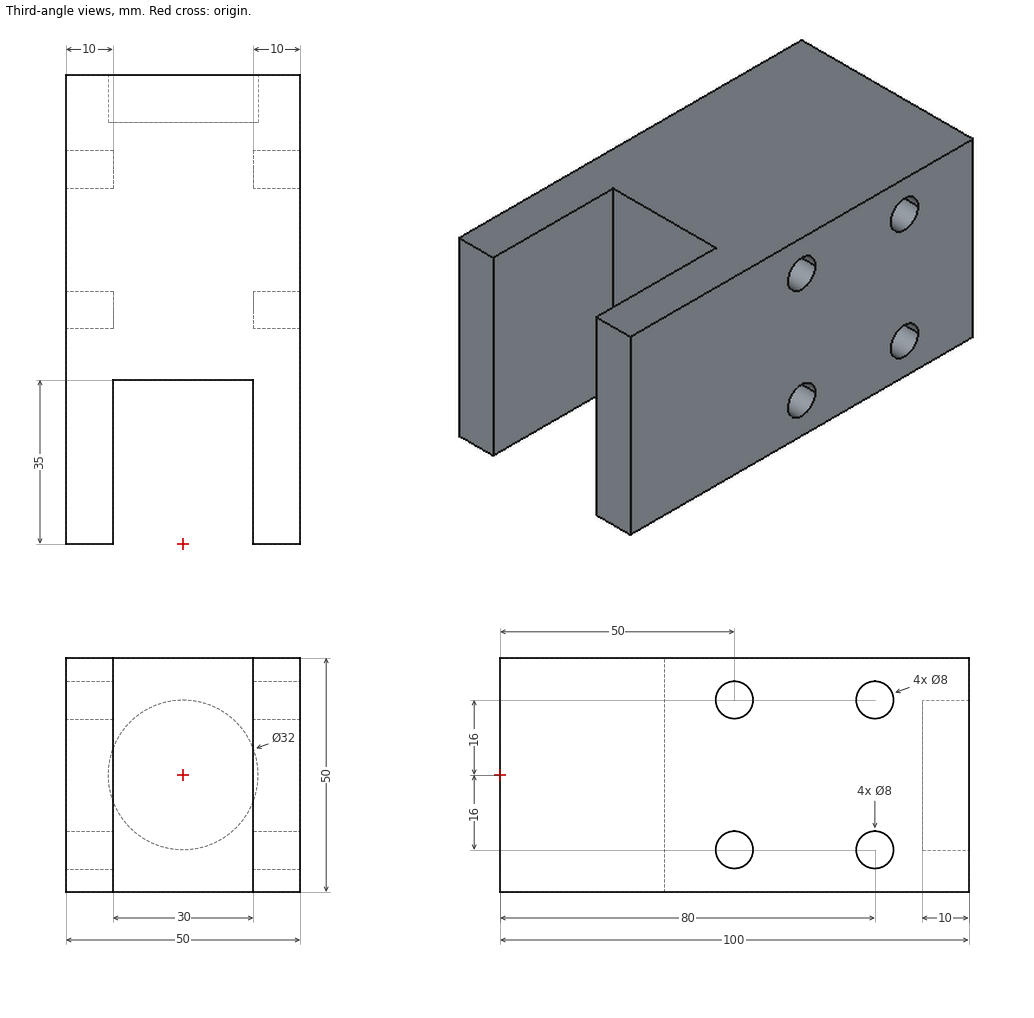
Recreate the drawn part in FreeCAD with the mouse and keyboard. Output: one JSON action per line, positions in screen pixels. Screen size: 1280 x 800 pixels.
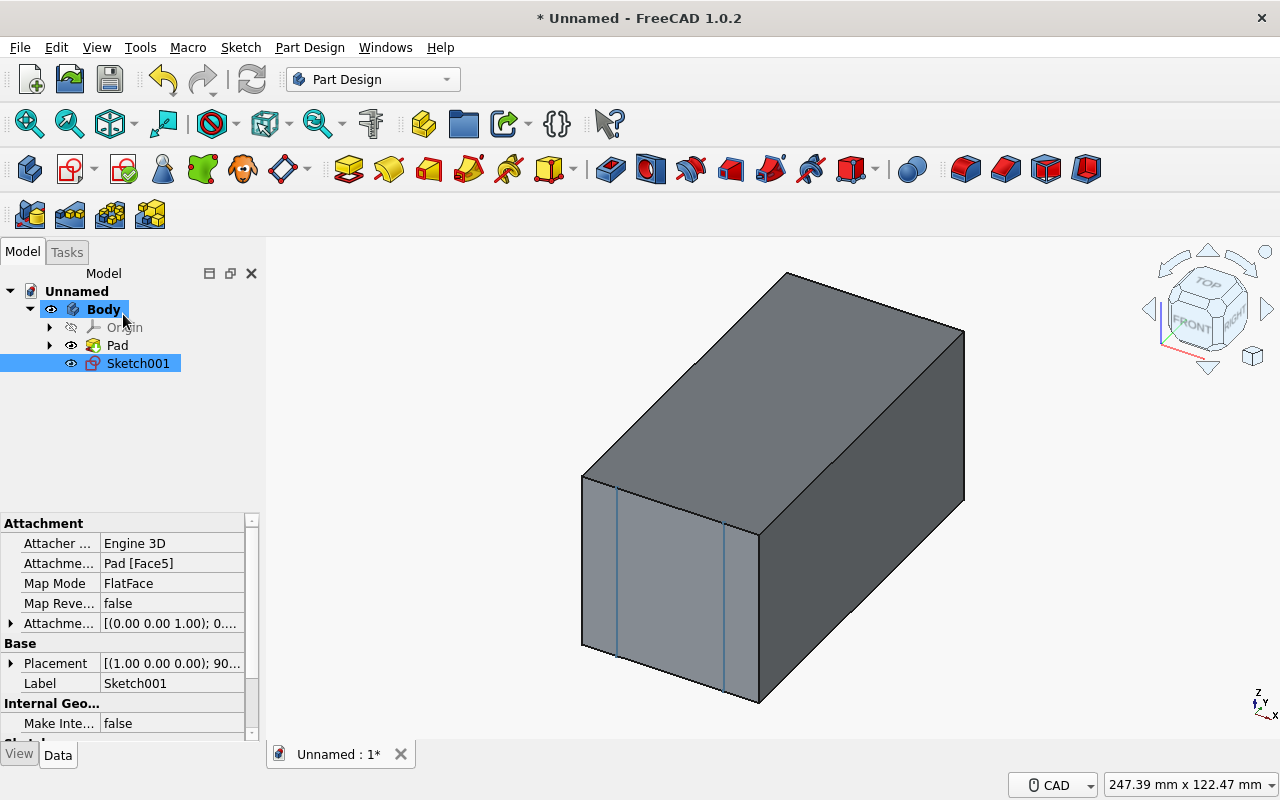
{"action": "left_click", "coordinate": [612, 170]}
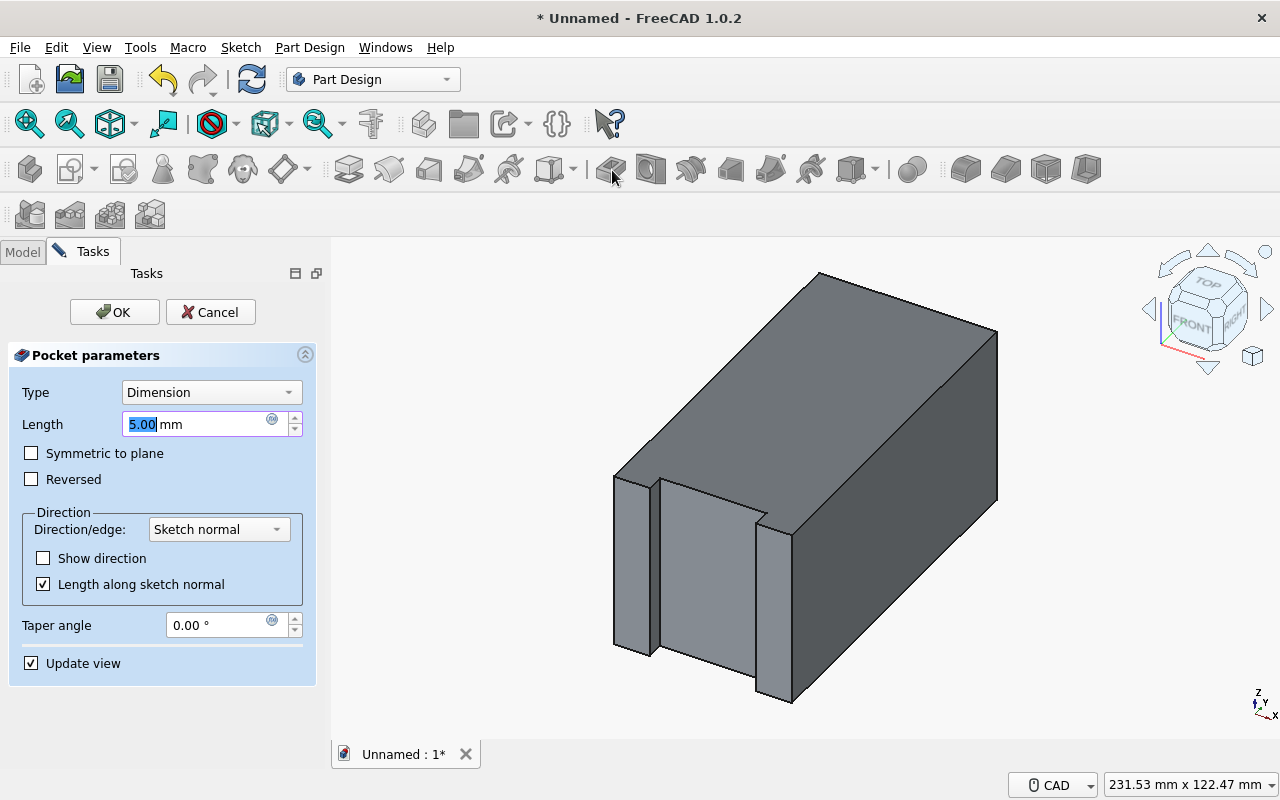
{"action": "type", "text": "35"}
{"action": "key", "text": "Tab"}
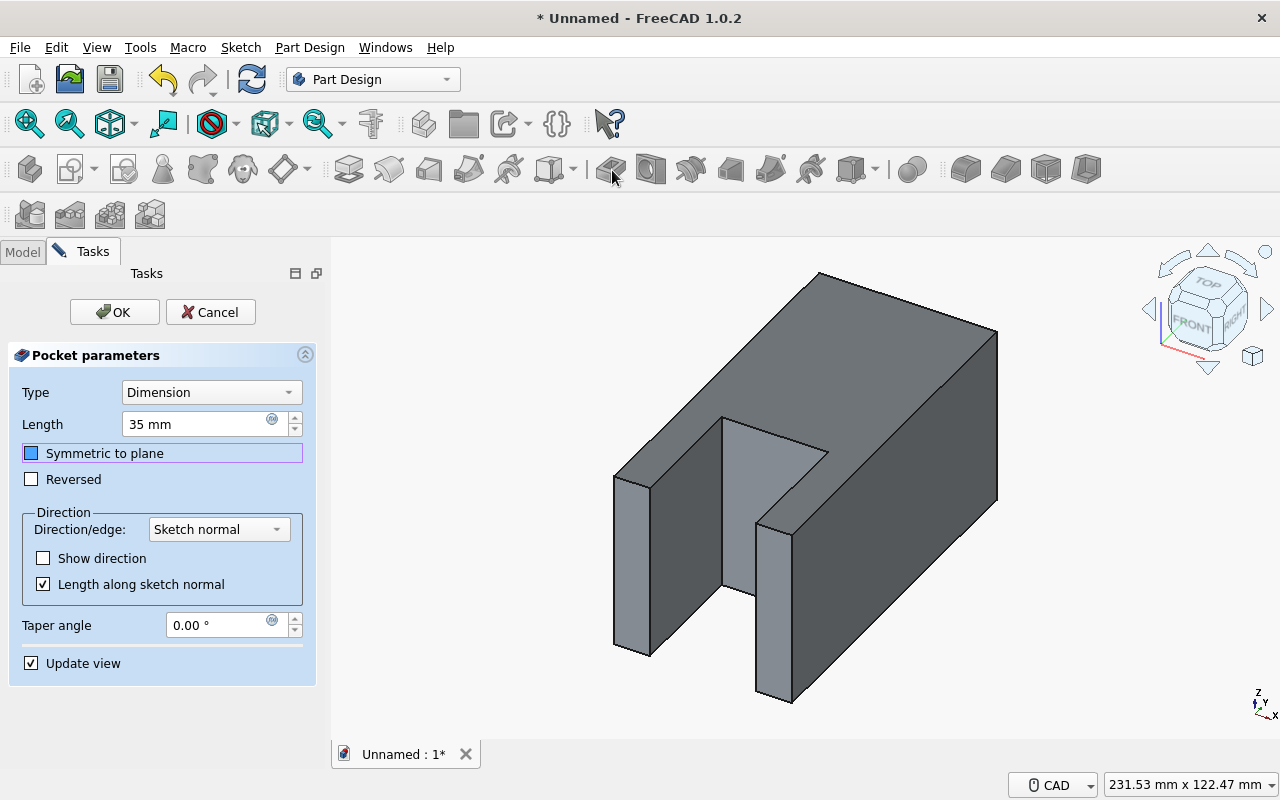
{"action": "left_click", "coordinate": [115, 312]}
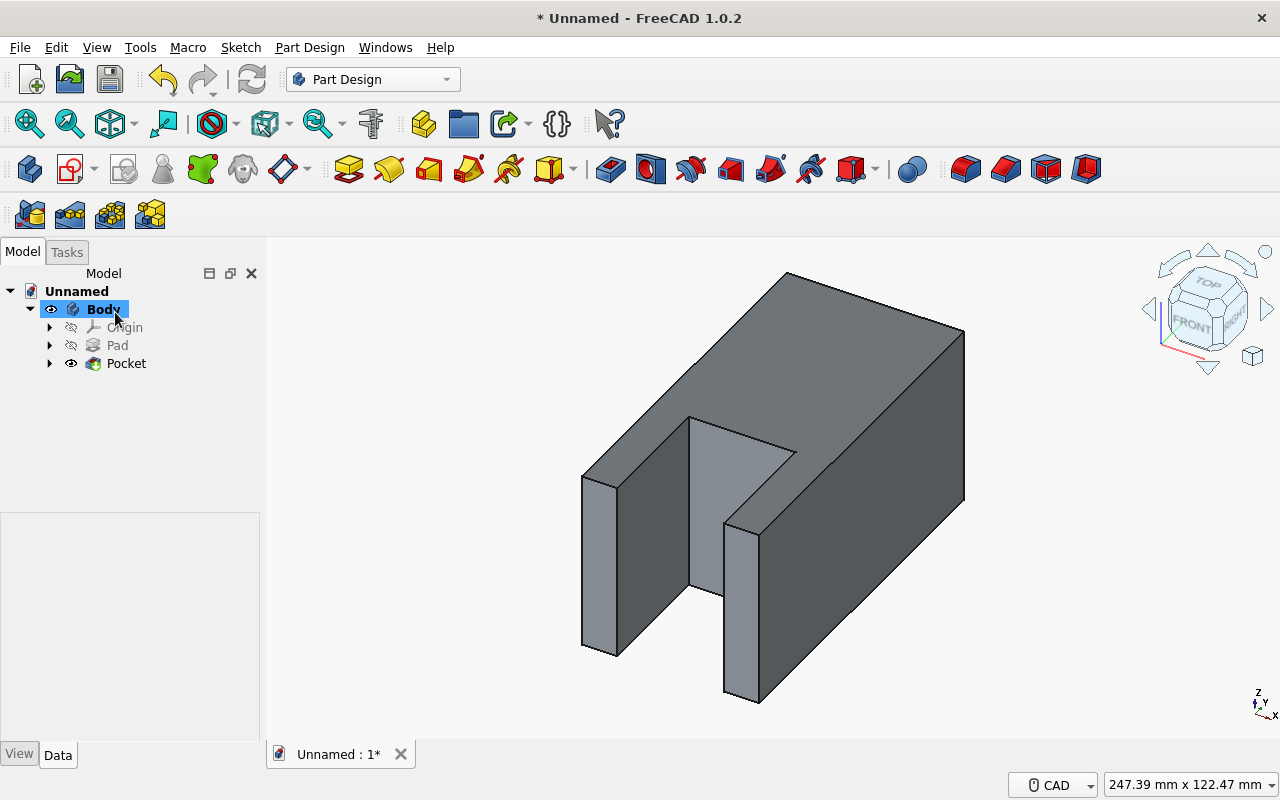
{"action": "key", "text": "4"}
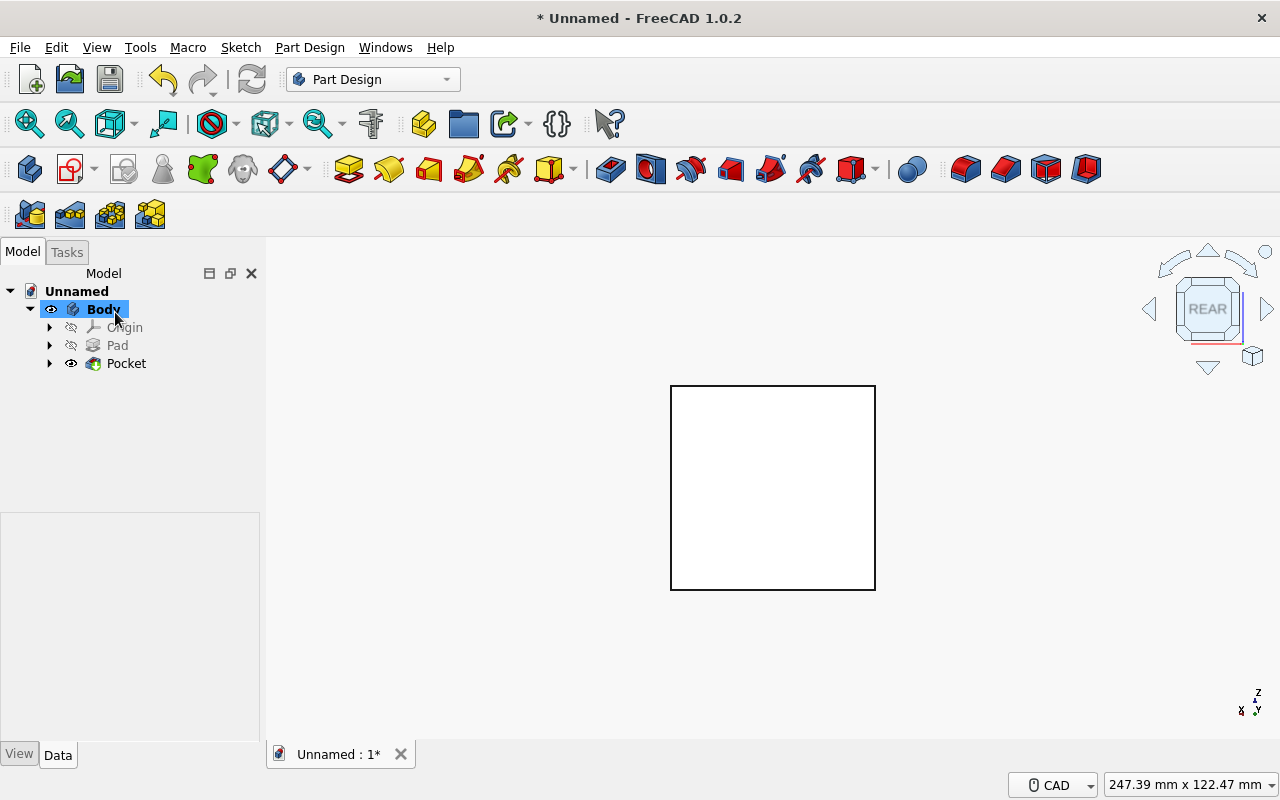
{"action": "left_click", "coordinate": [30, 124]}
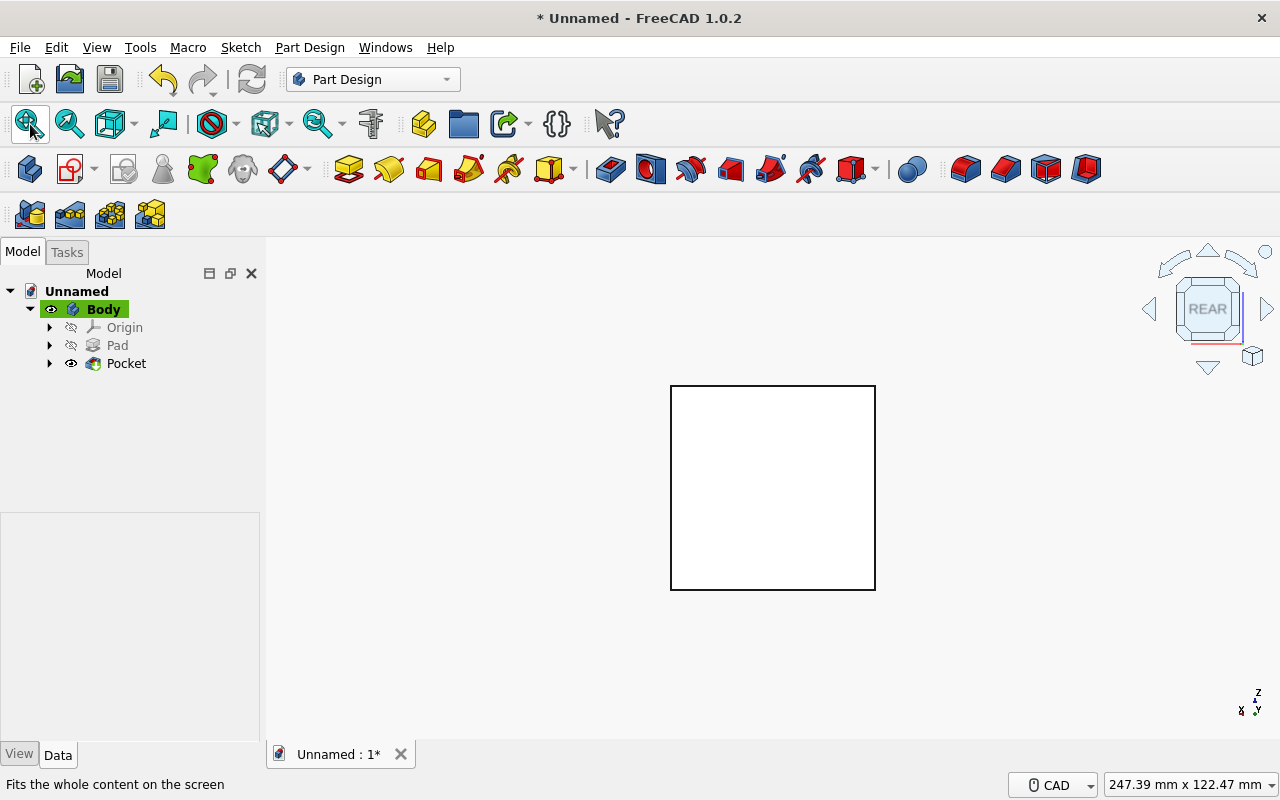
{"action": "left_click", "coordinate": [773, 487]}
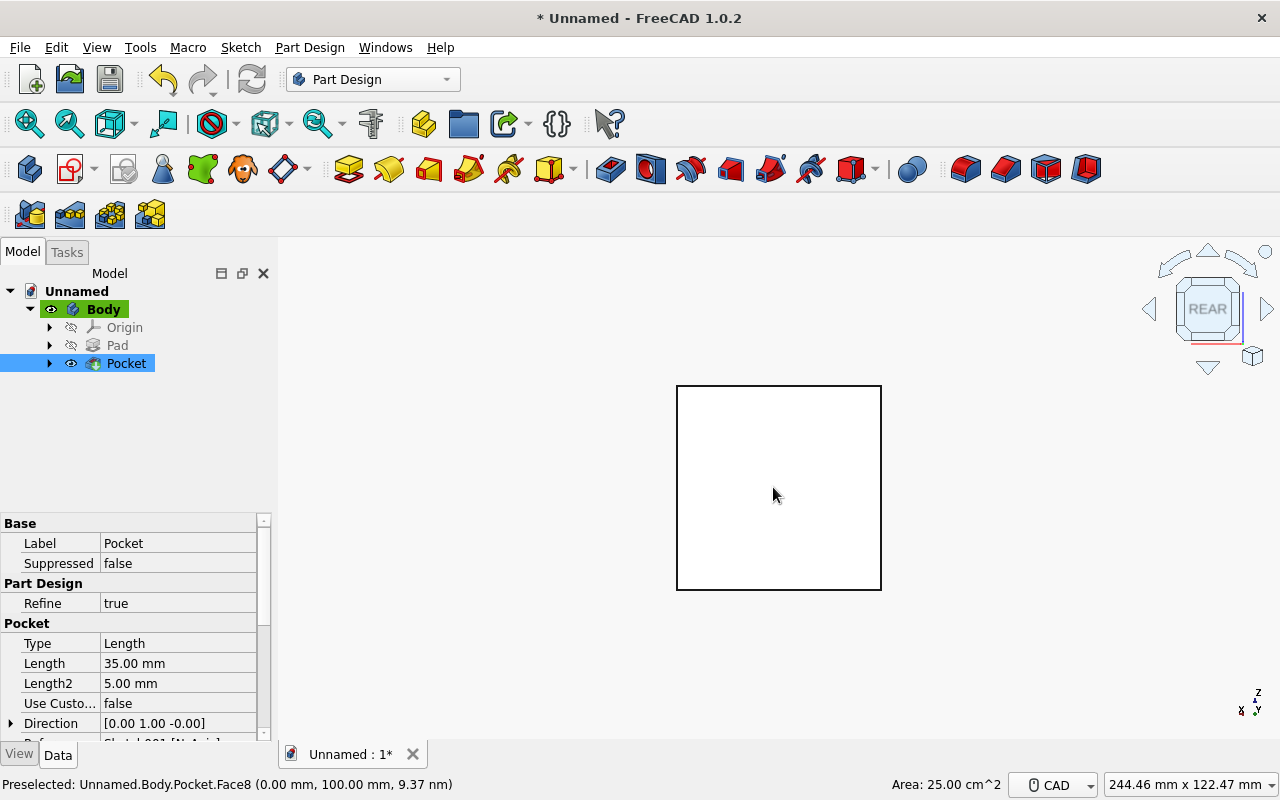
{"action": "left_click", "coordinate": [70, 170]}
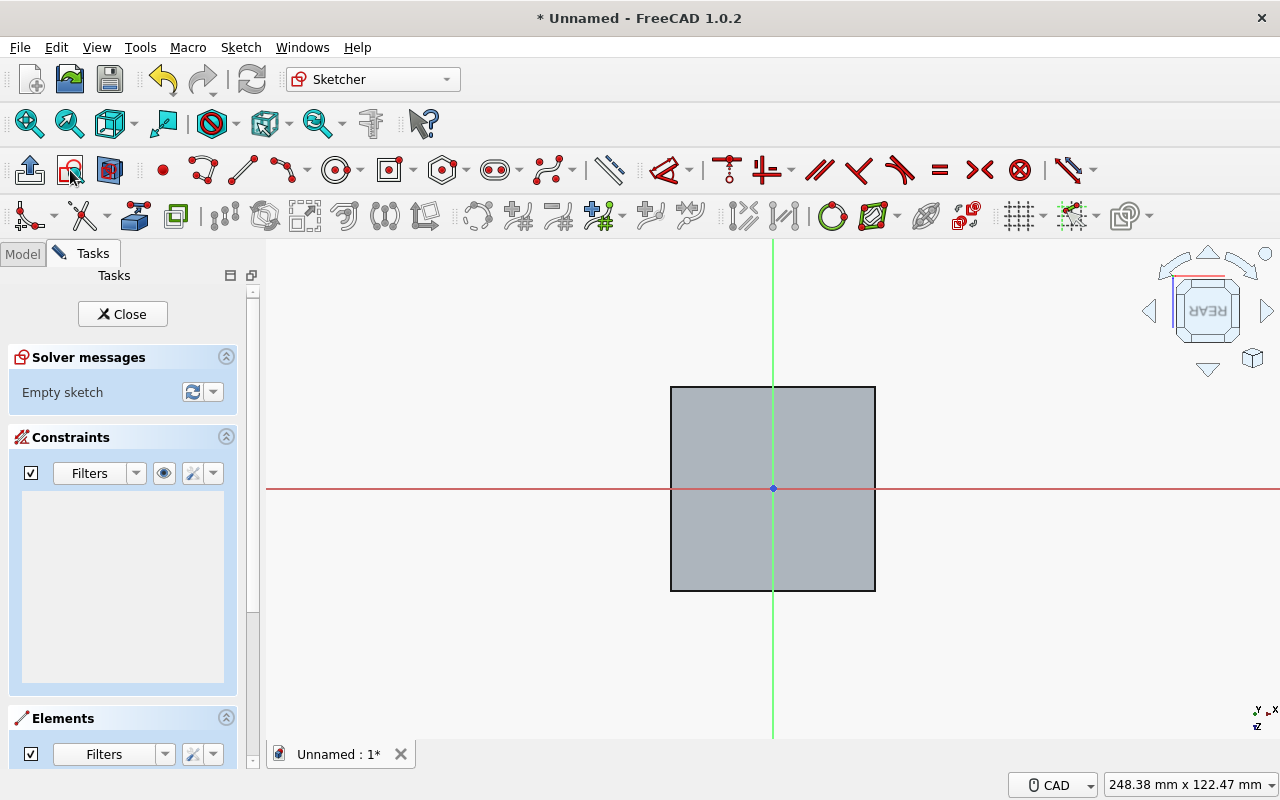
{"action": "scroll", "coordinate": [829, 489], "scroll_direction": "up", "scroll_amount": 4}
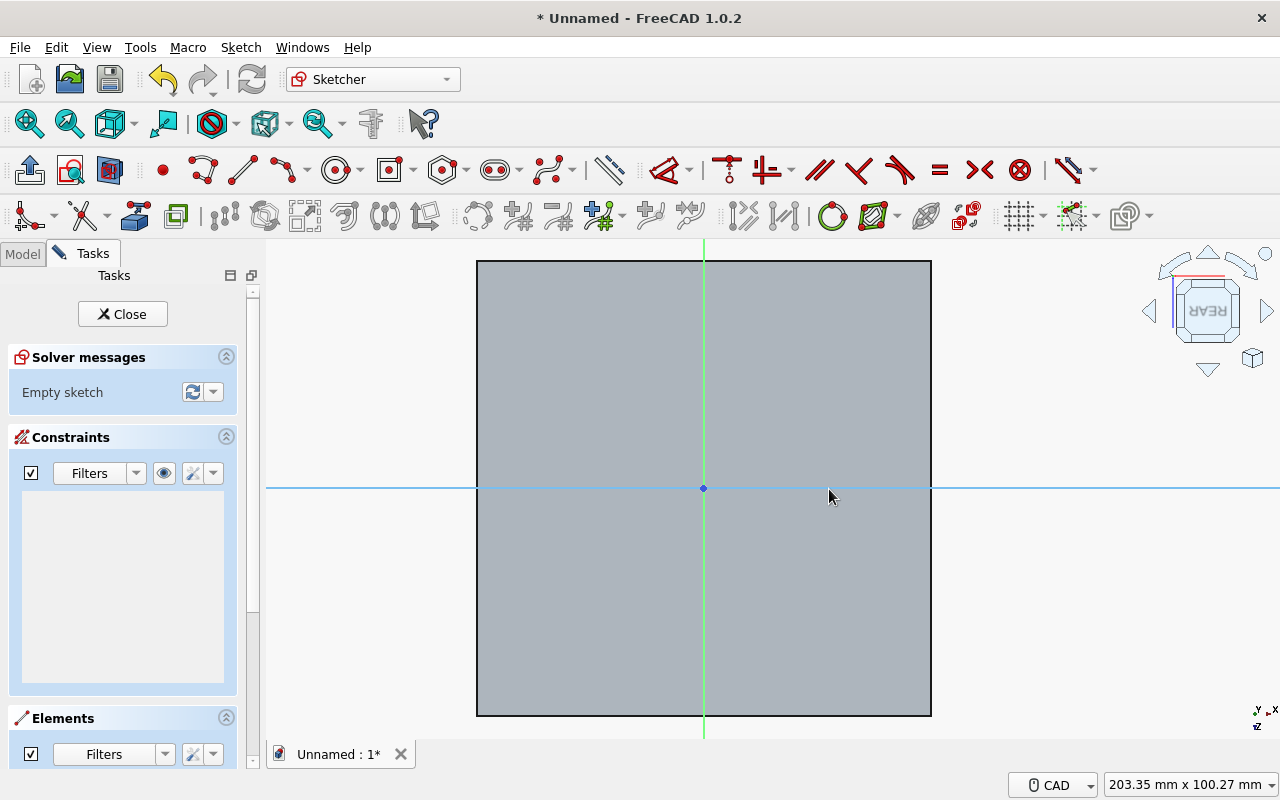
{"action": "left_click", "coordinate": [336, 170]}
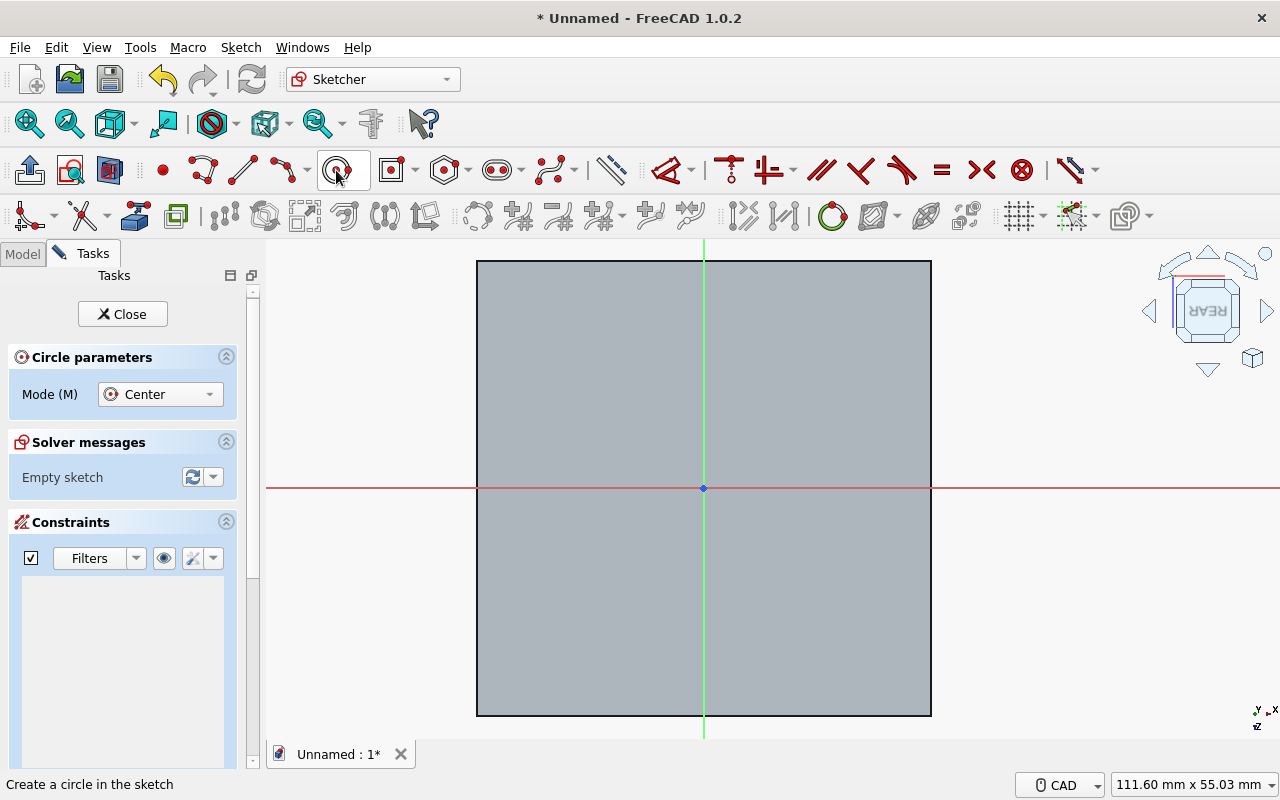
{"action": "left_click", "coordinate": [704, 488]}
{"action": "mouse_move", "coordinate": [806, 386]}